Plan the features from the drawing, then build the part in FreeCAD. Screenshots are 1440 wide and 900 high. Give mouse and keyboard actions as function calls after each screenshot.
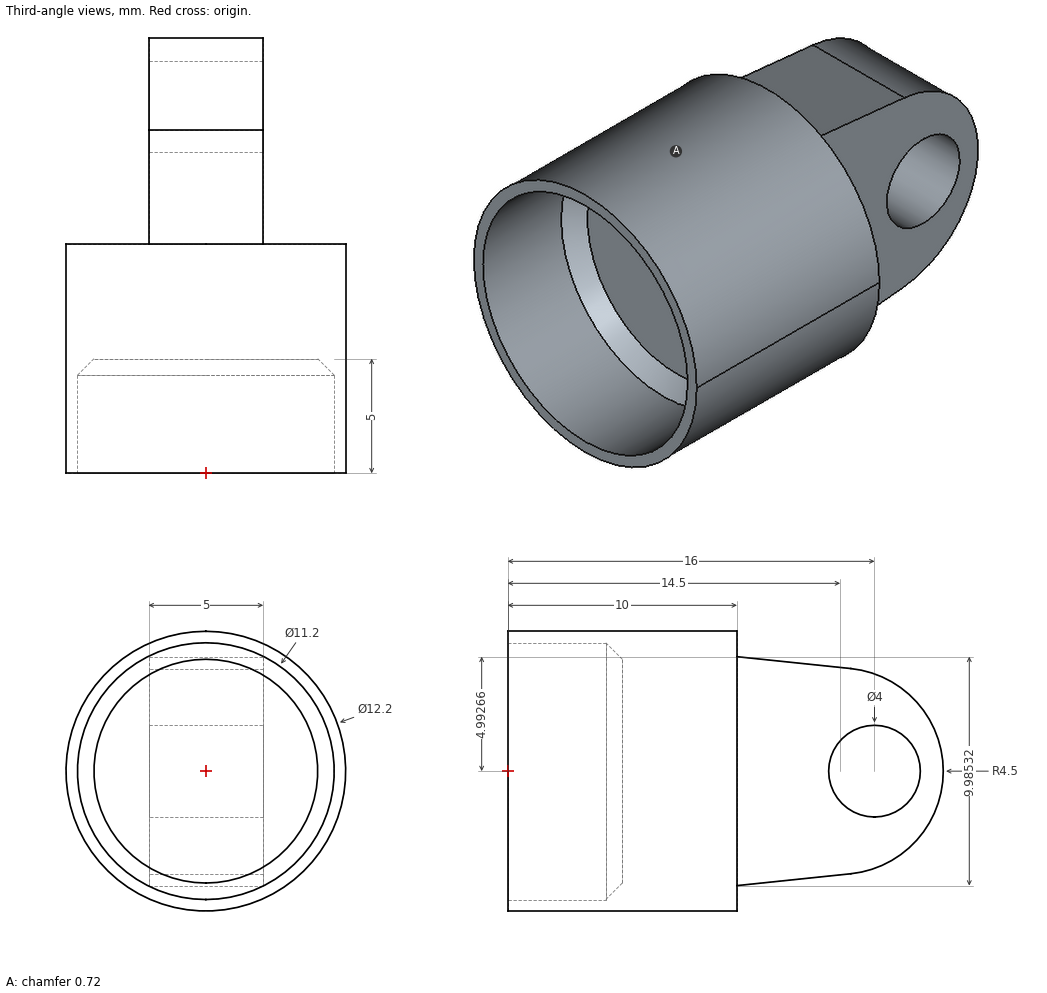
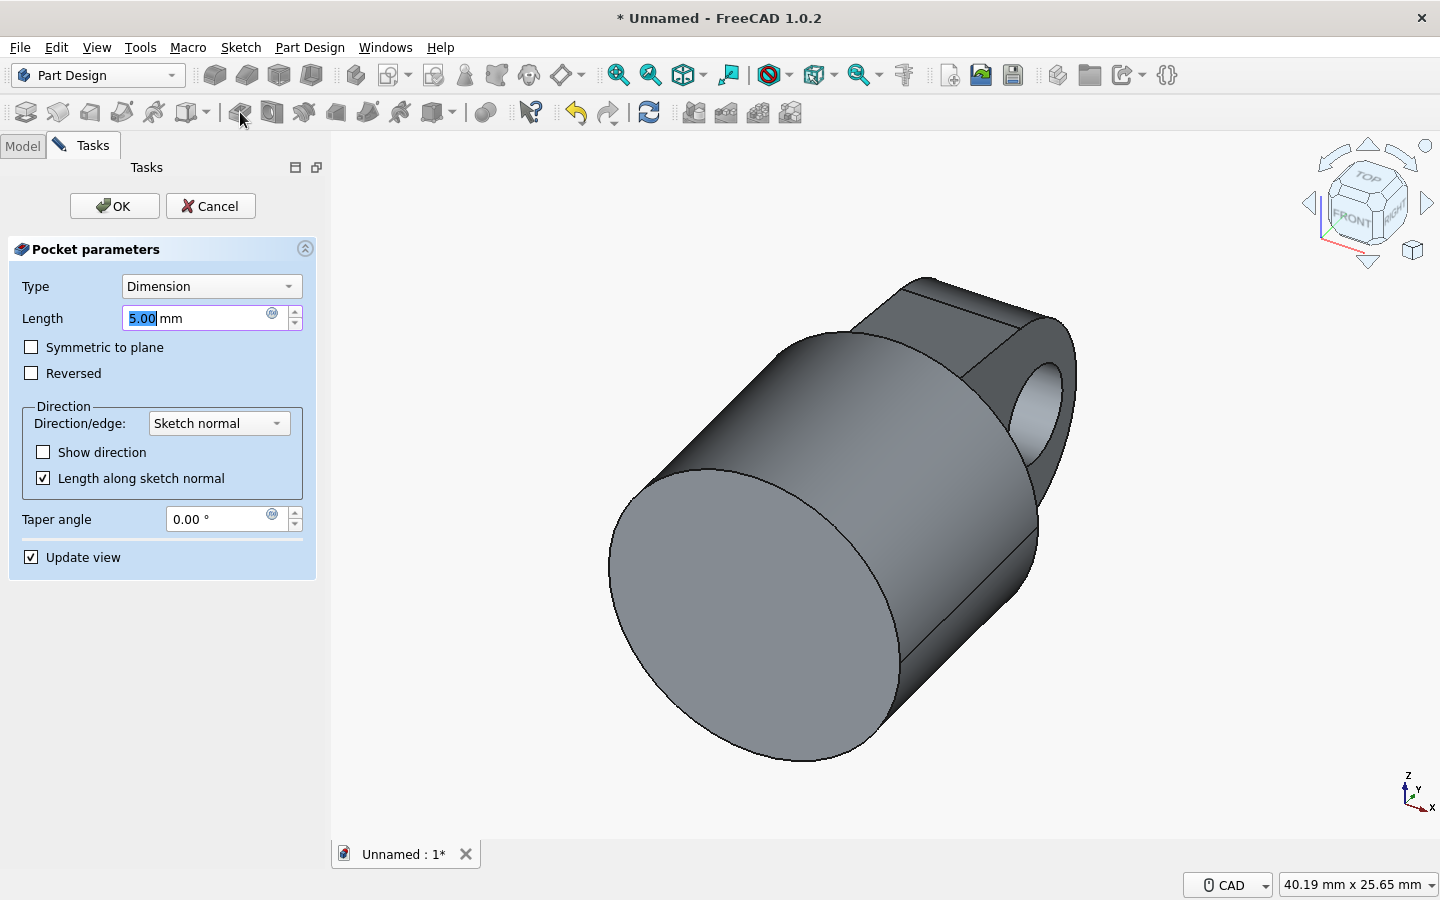
click(212, 286)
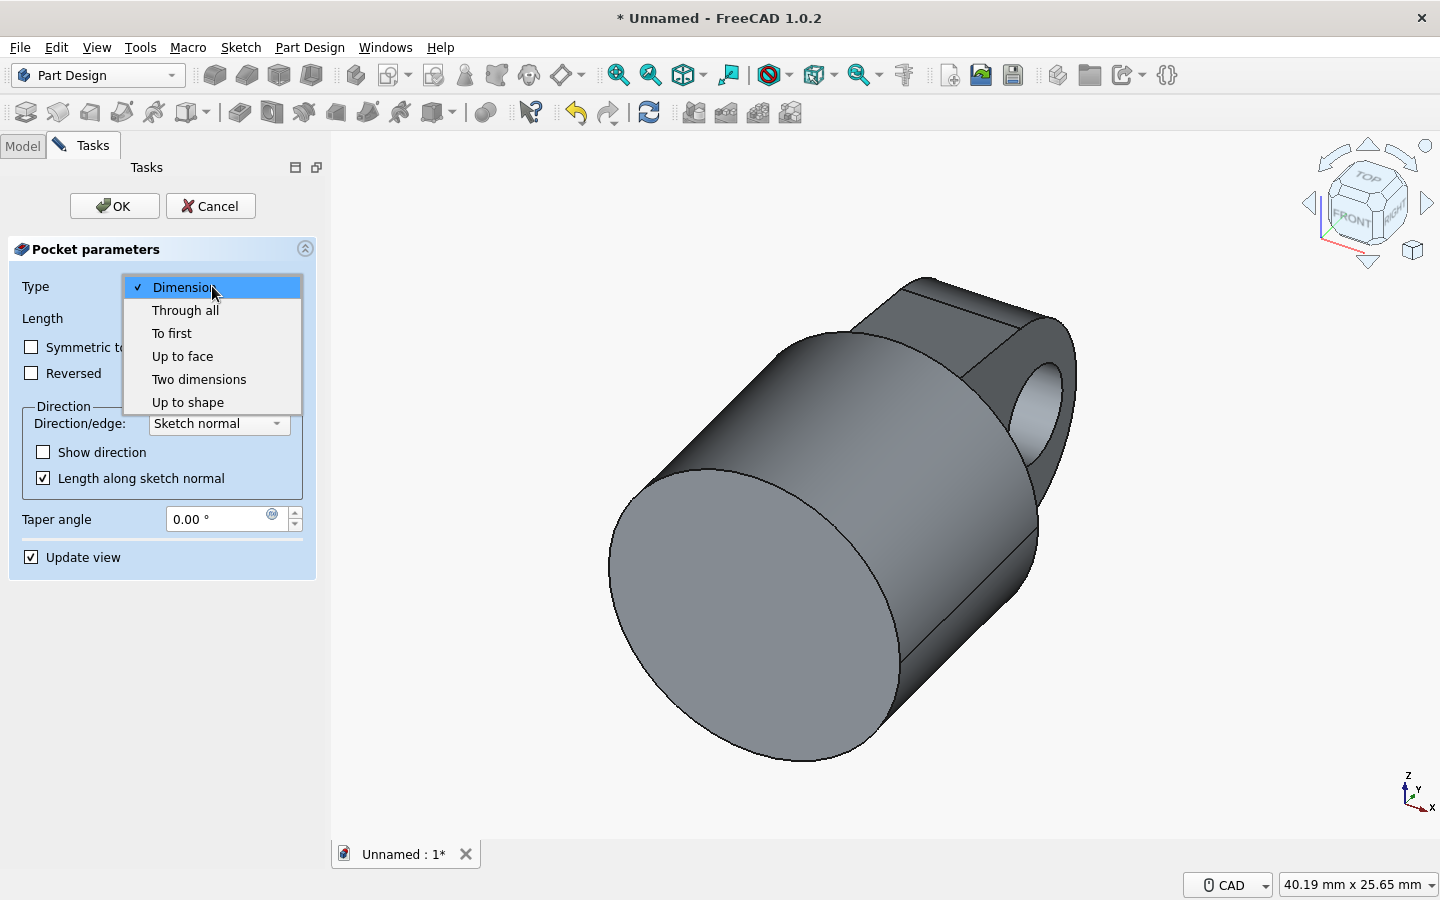
click(212, 310)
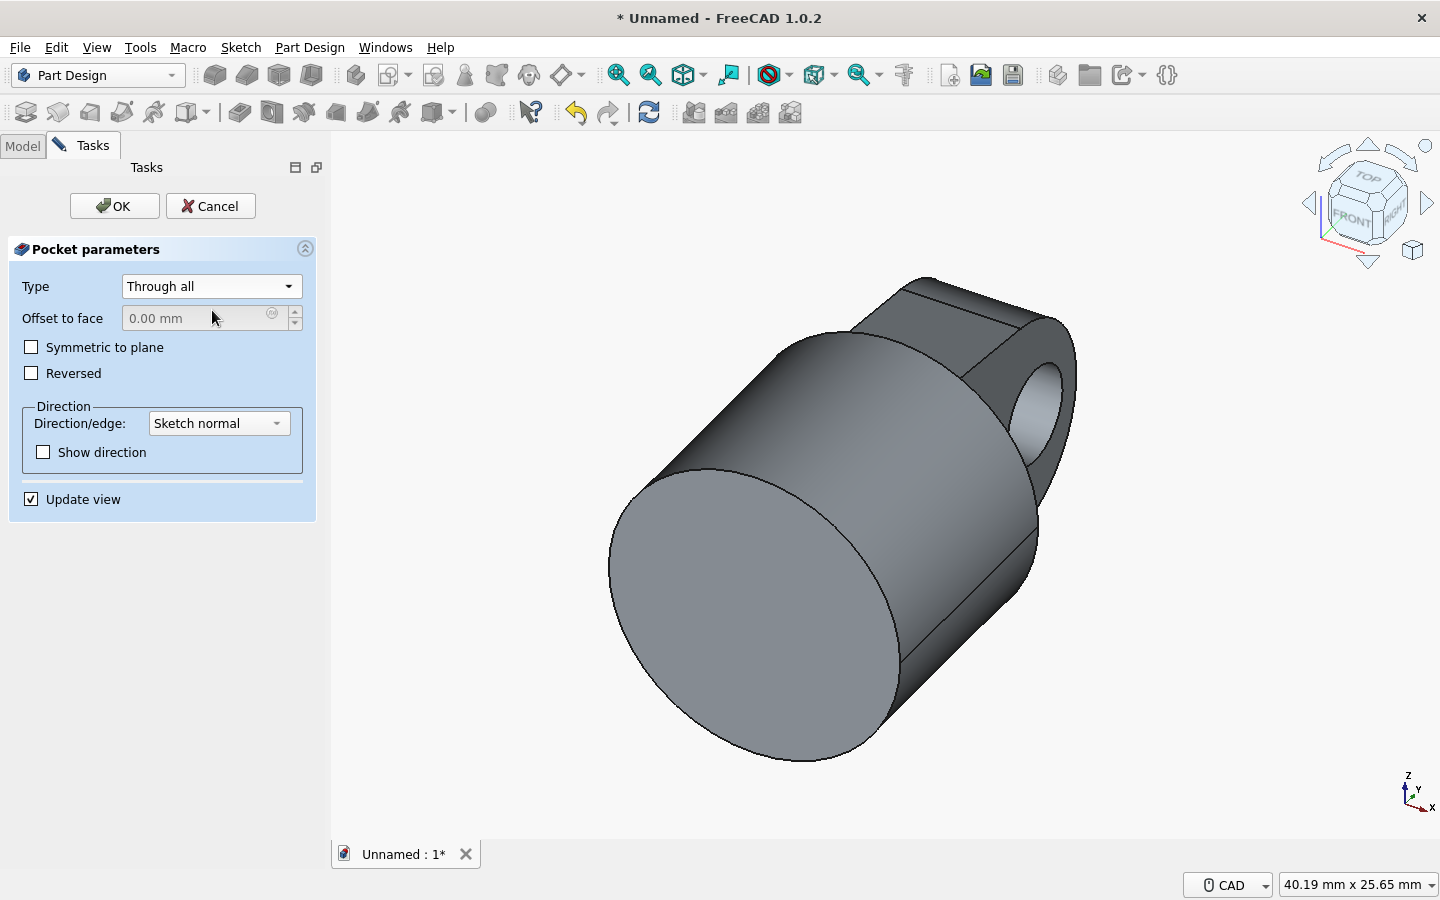
click(115, 206)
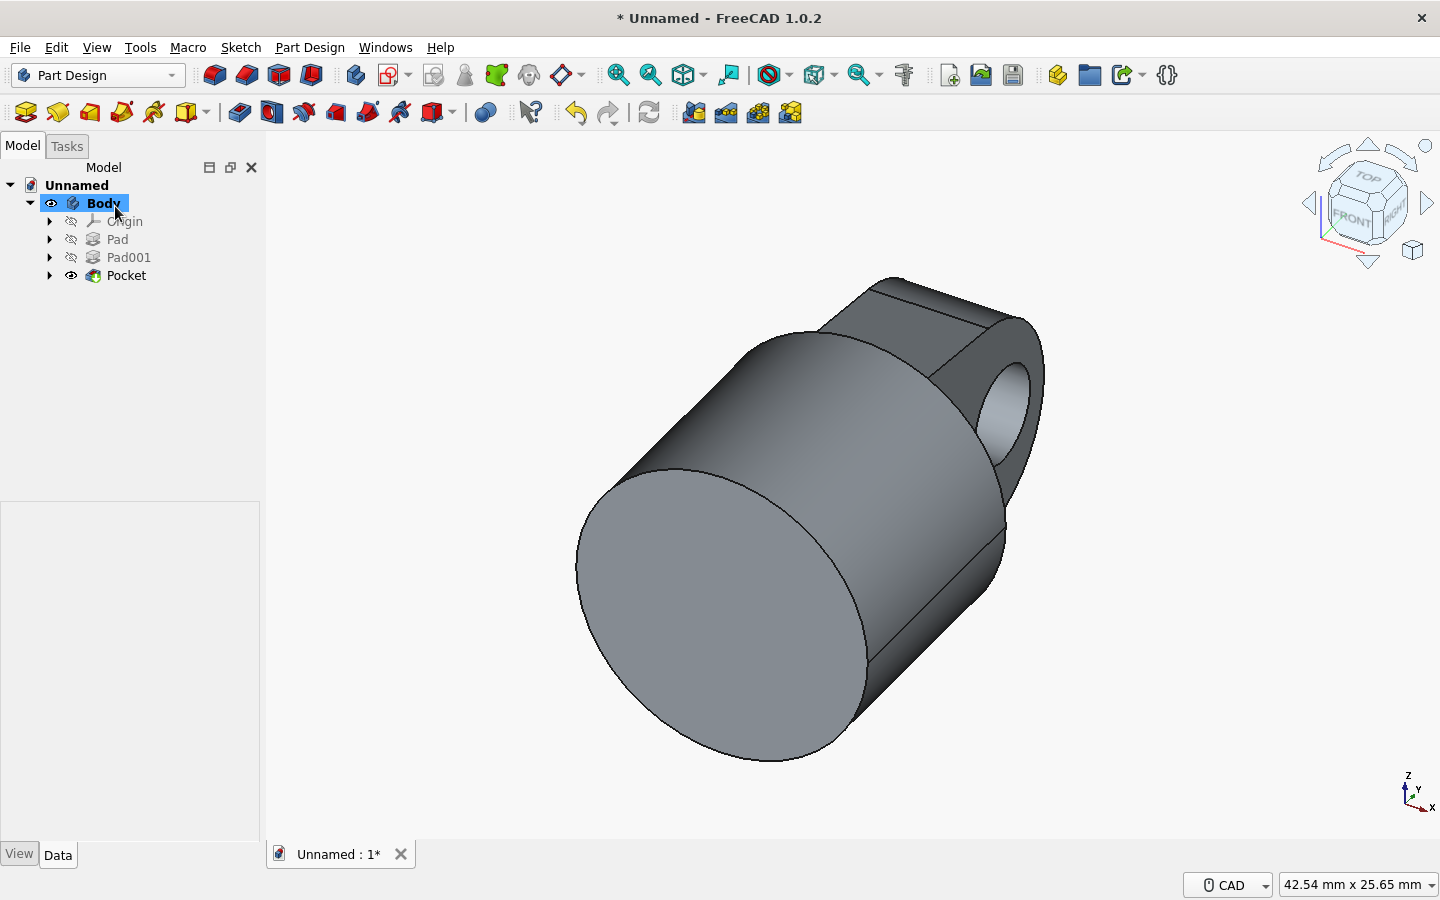
click(722, 614)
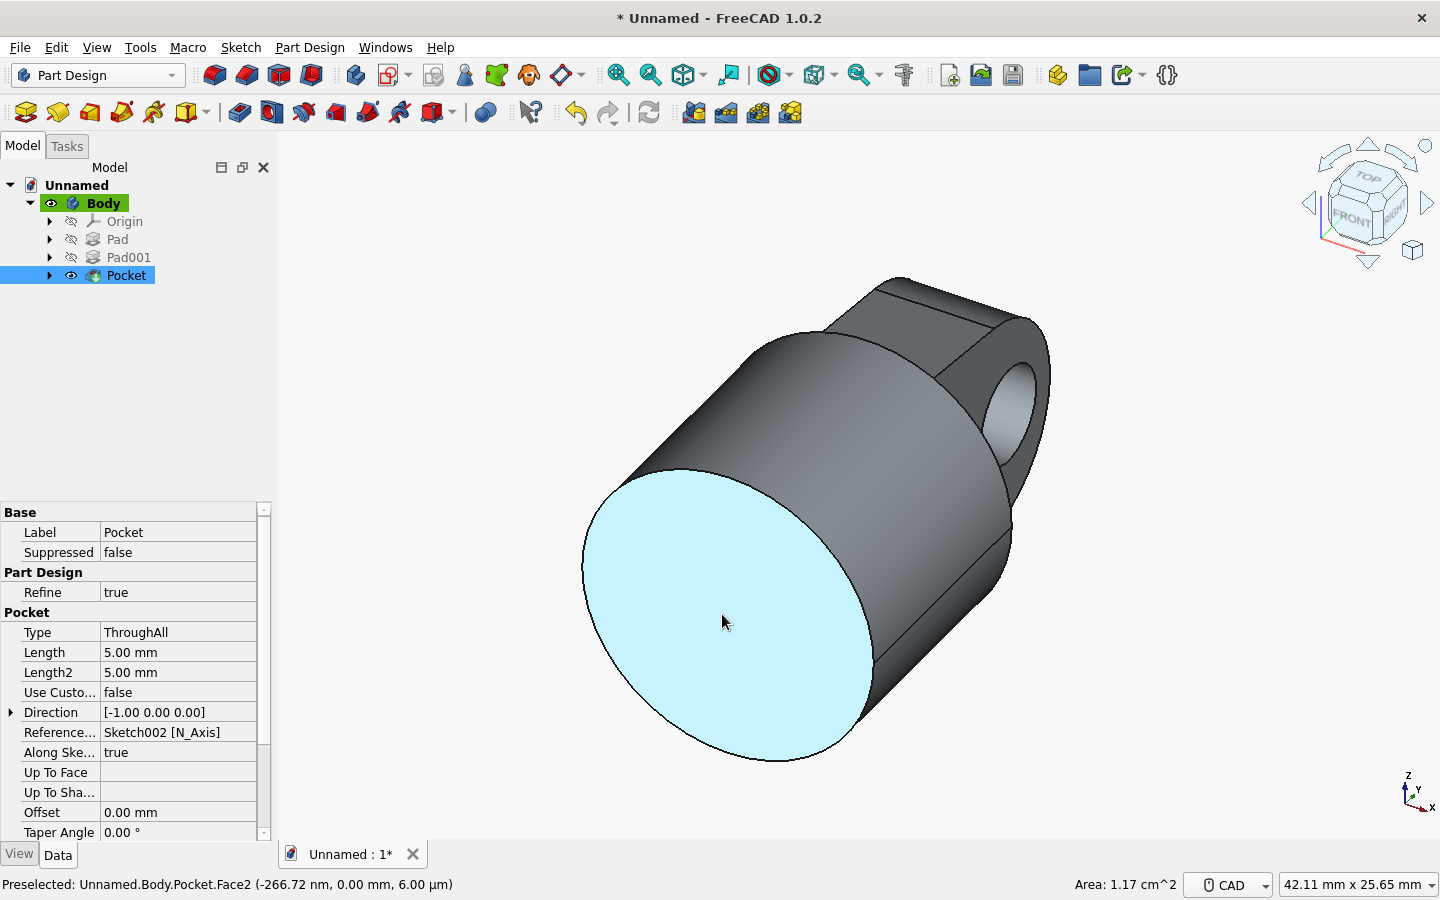
click(388, 76)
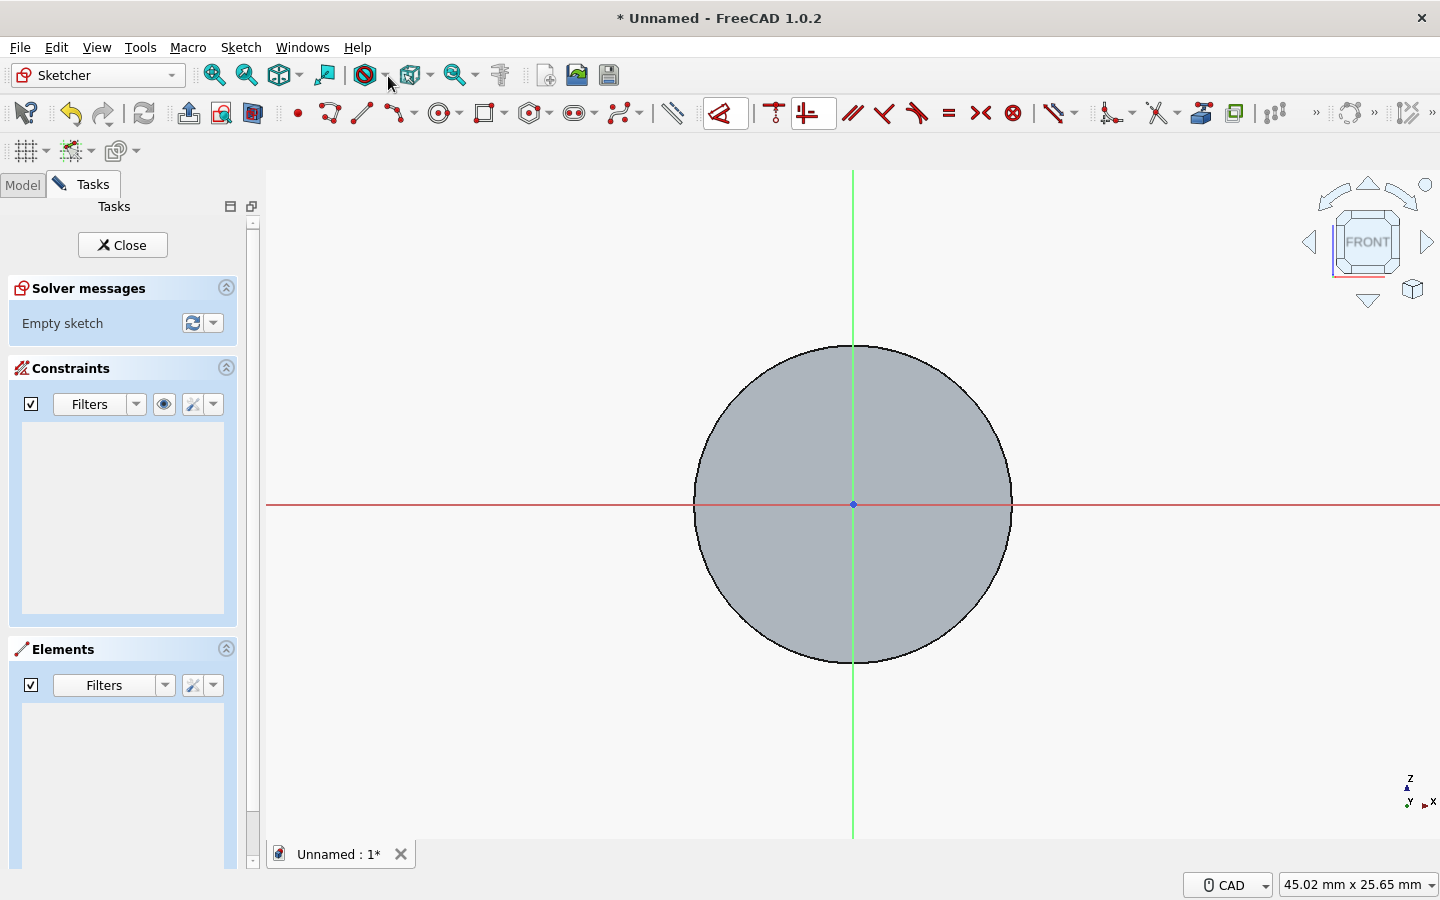
scroll(992, 505, up, 2)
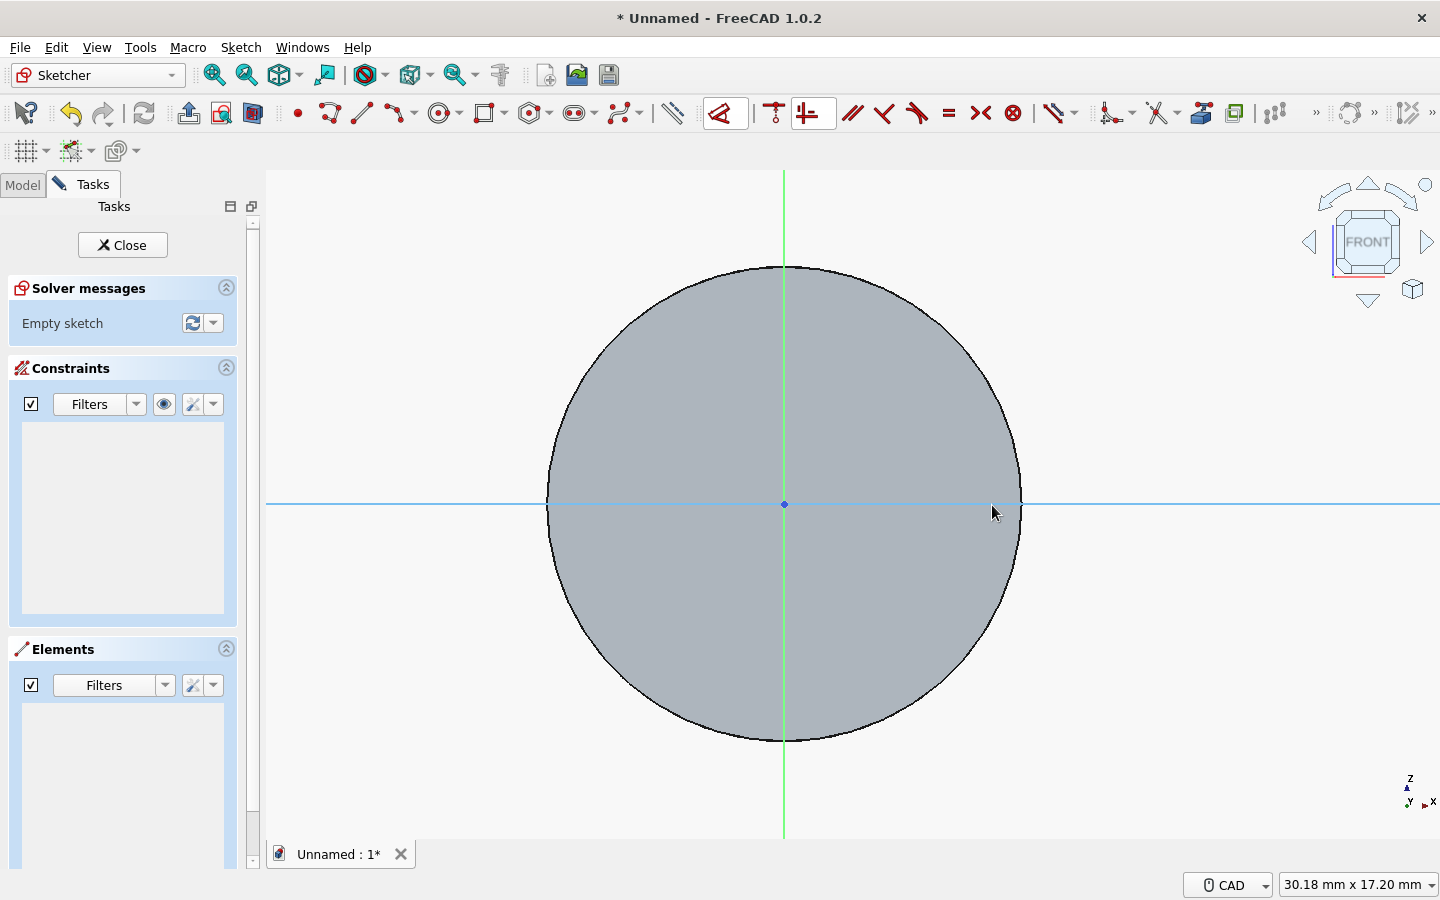
click(440, 114)